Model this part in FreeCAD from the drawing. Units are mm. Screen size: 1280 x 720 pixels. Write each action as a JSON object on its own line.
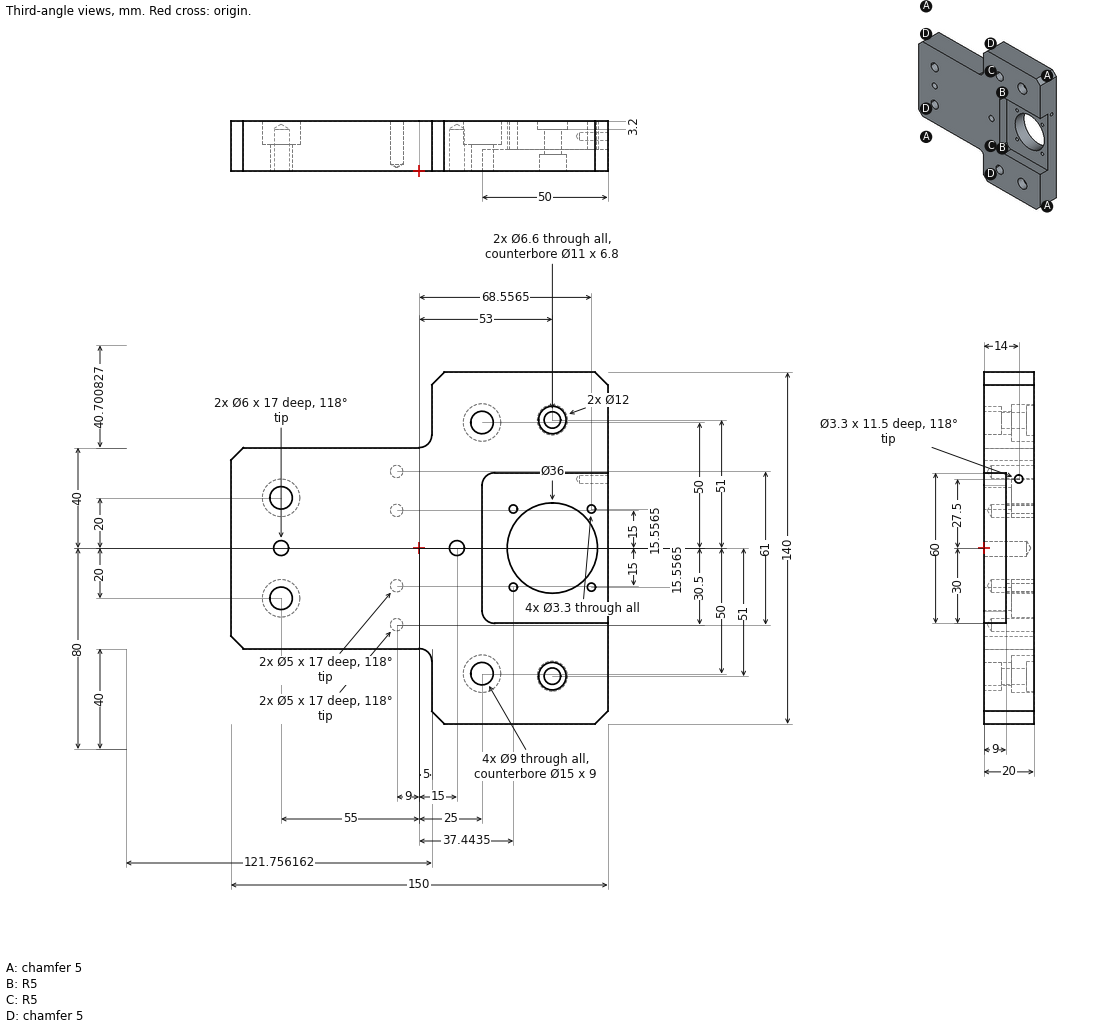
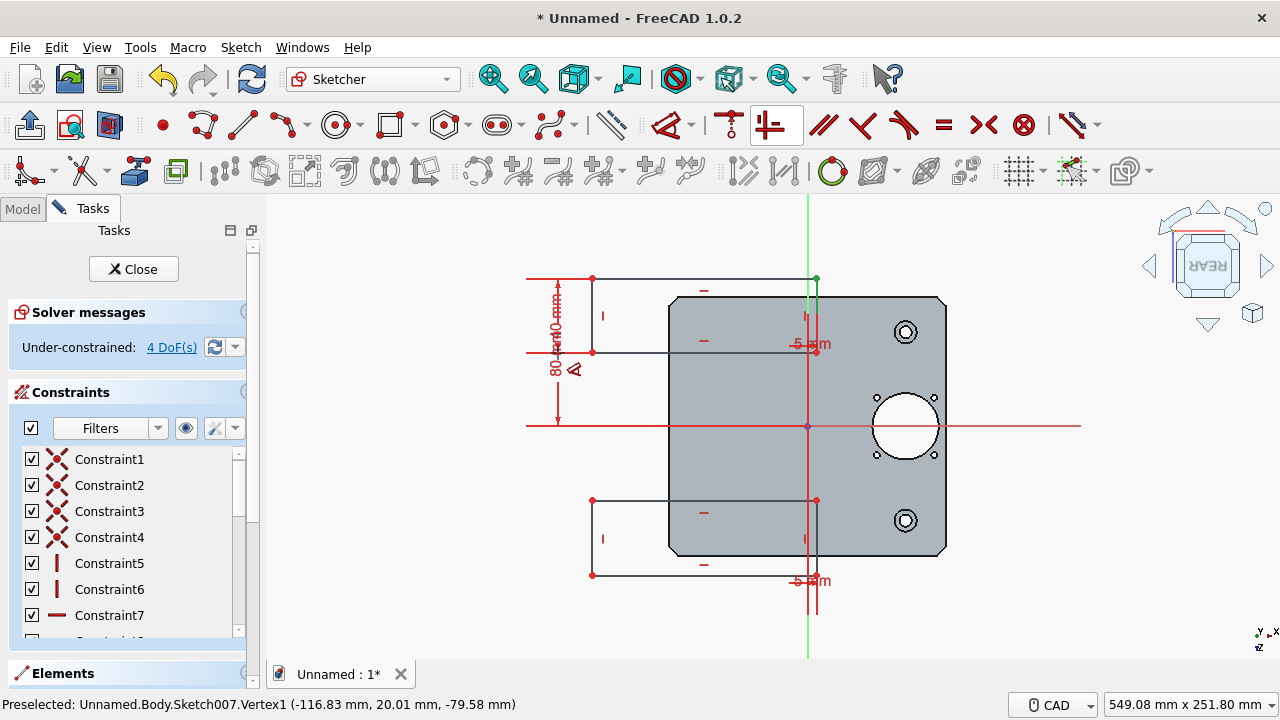
{"action": "left_click", "coordinate": [592, 501]}
{"action": "left_click", "coordinate": [558, 464]}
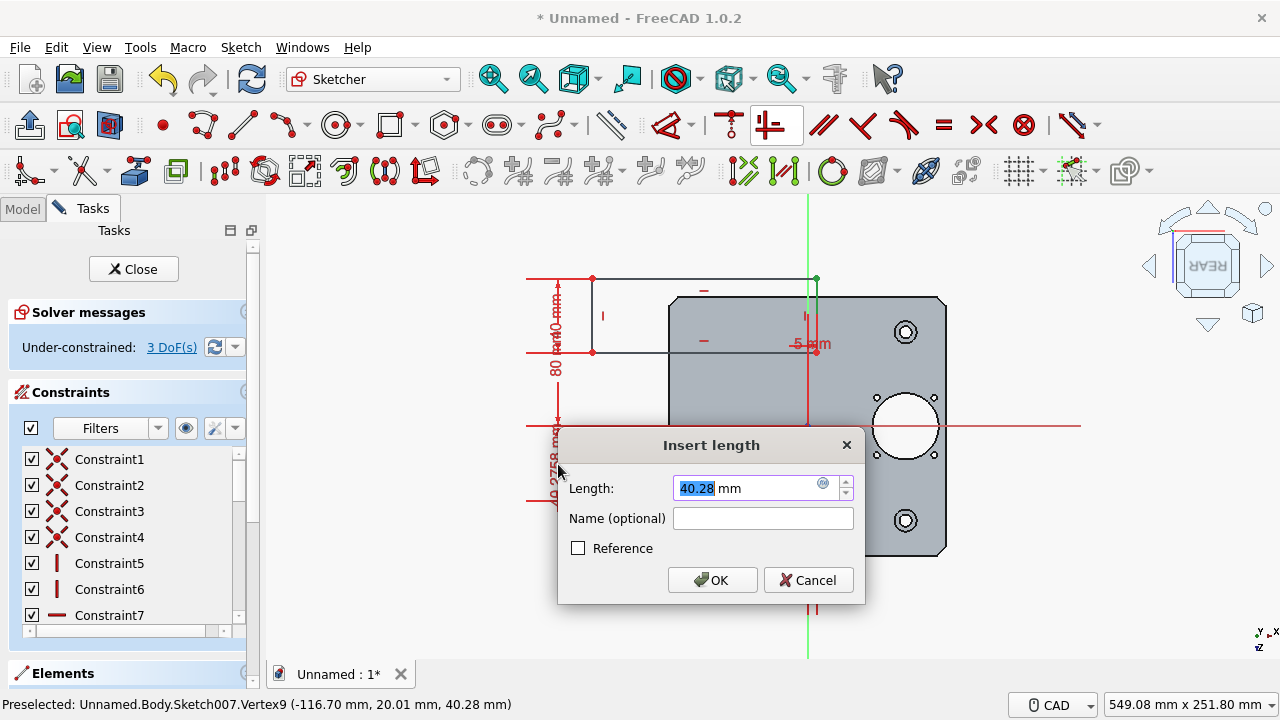
{"action": "type", "text": "40"}
{"action": "key", "text": "Return"}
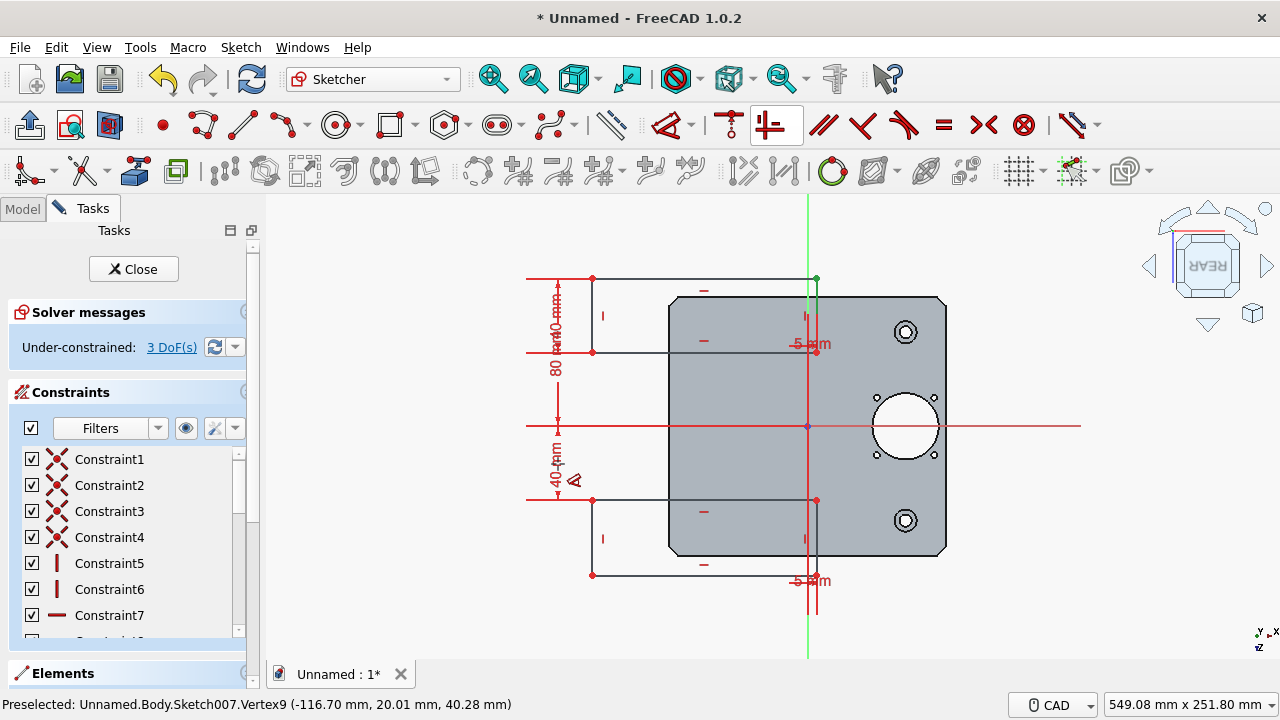
{"action": "left_click", "coordinate": [592, 523]}
{"action": "left_click", "coordinate": [558, 538]}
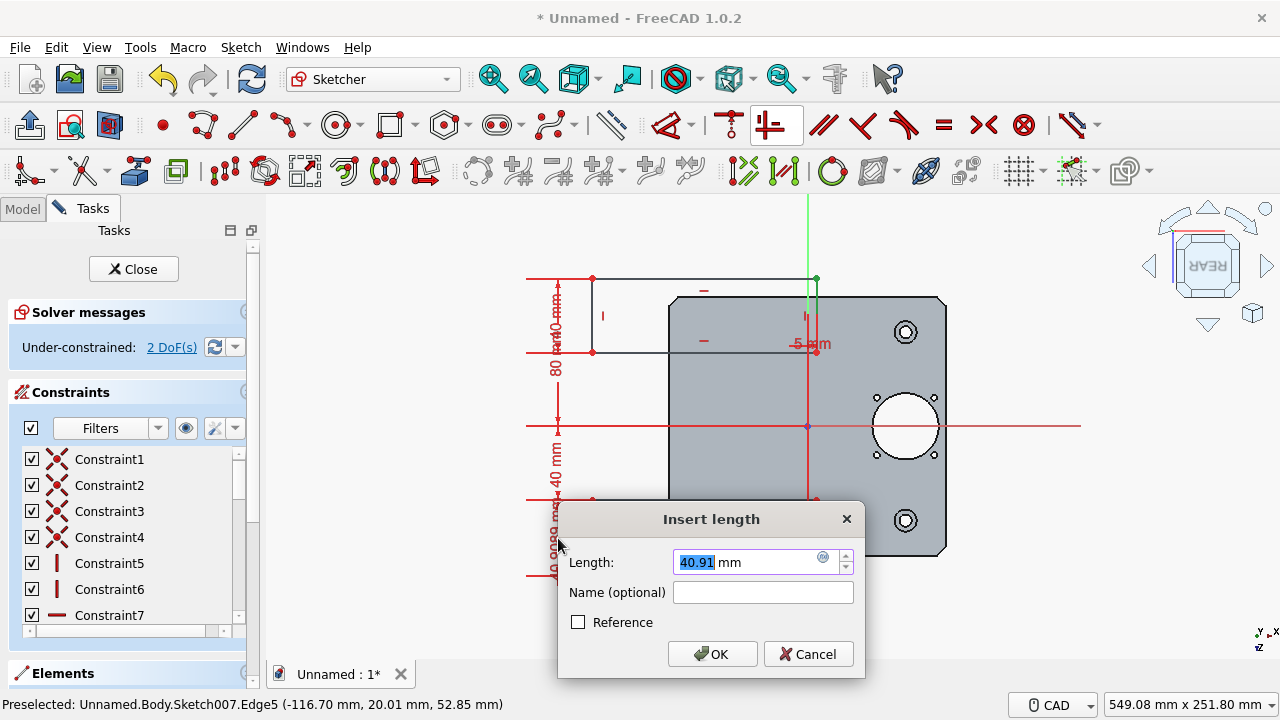
{"action": "type", "text": "40.700827"}
{"action": "key", "text": "Return"}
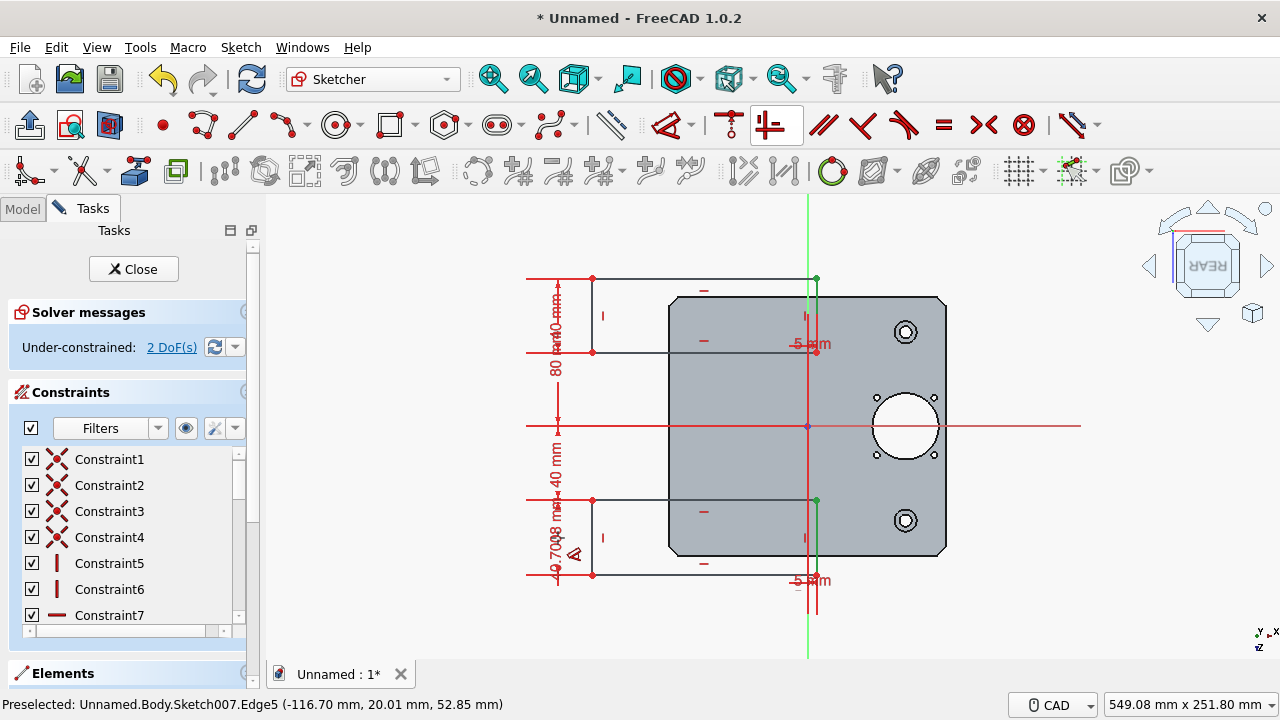
{"action": "left_click", "coordinate": [659, 353]}
{"action": "left_click", "coordinate": [704, 319]}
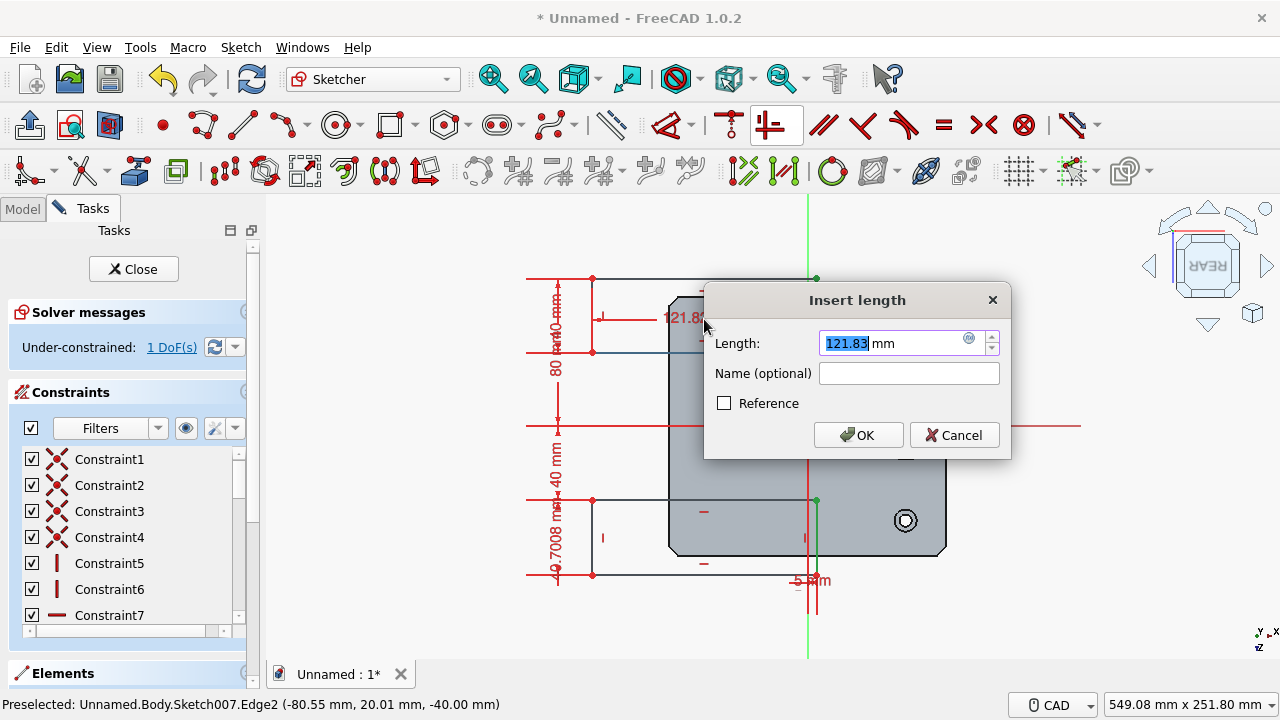
{"action": "type", "text": "121.756162"}
{"action": "key", "text": "Return"}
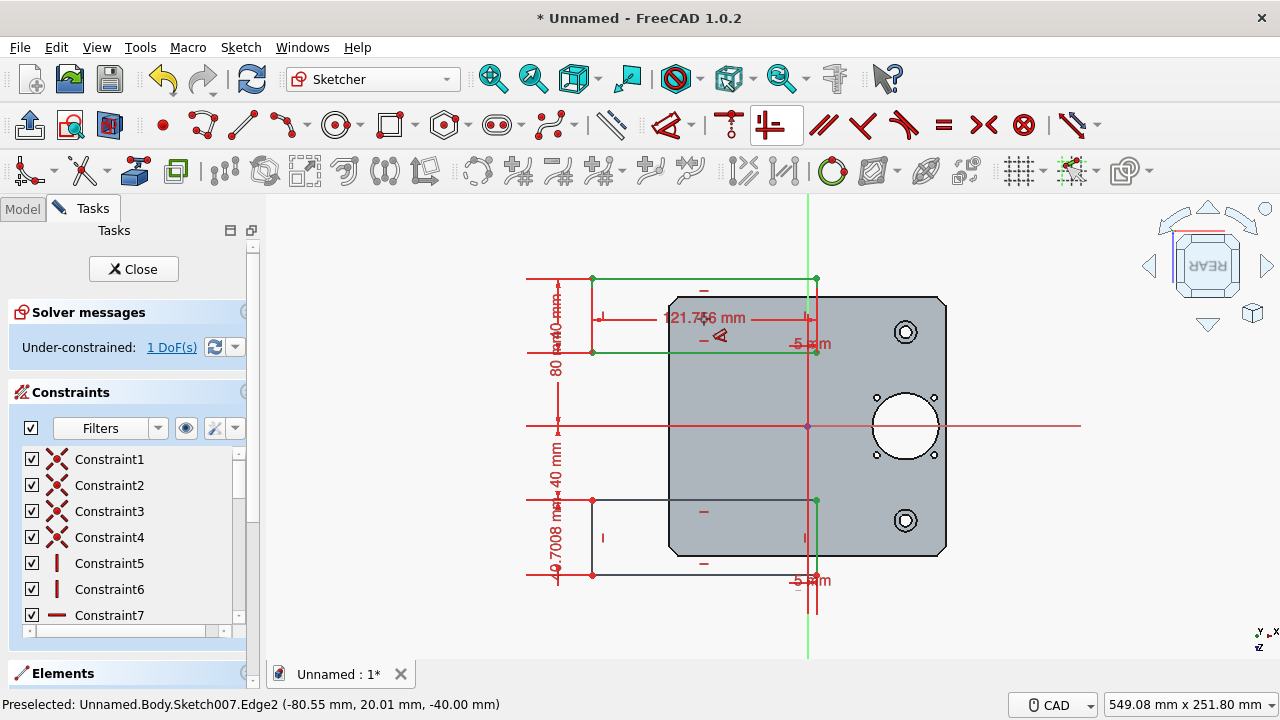
{"action": "left_click", "coordinate": [660, 575]}
{"action": "left_click", "coordinate": [705, 609]}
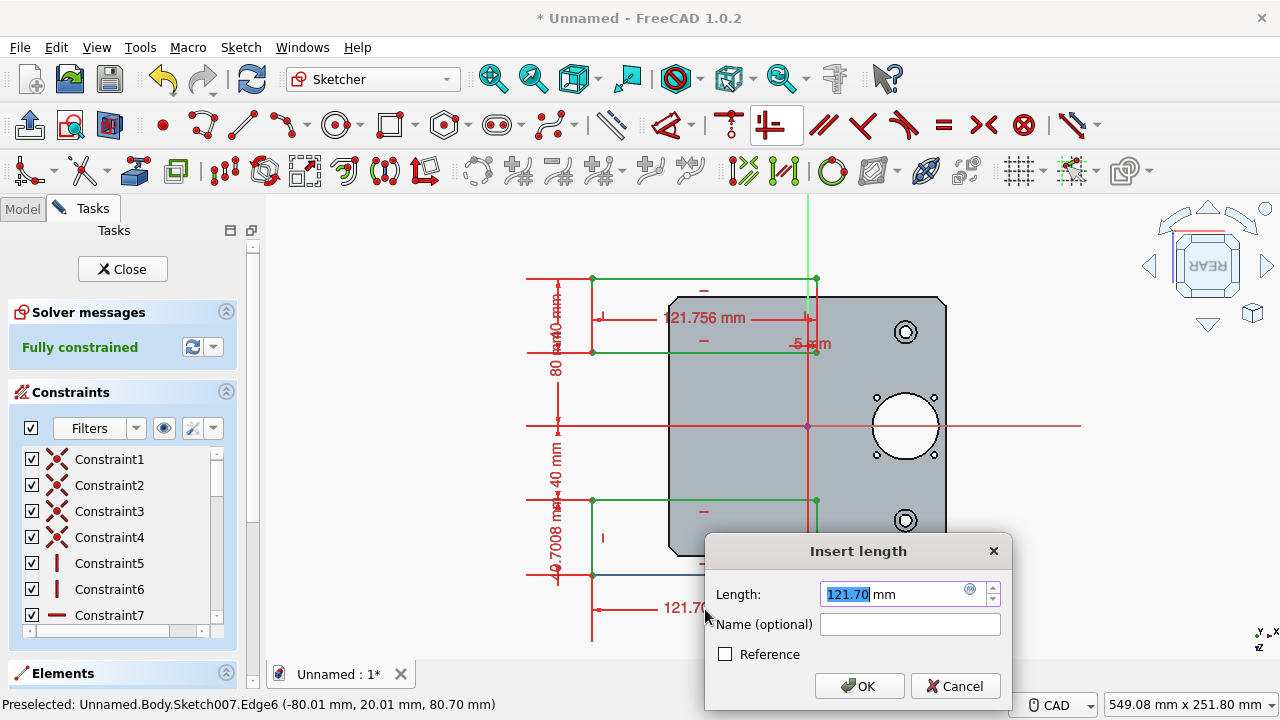
{"action": "type", "text": "121.756162"}
{"action": "key", "text": "Return"}
{"action": "key", "text": "Escape"}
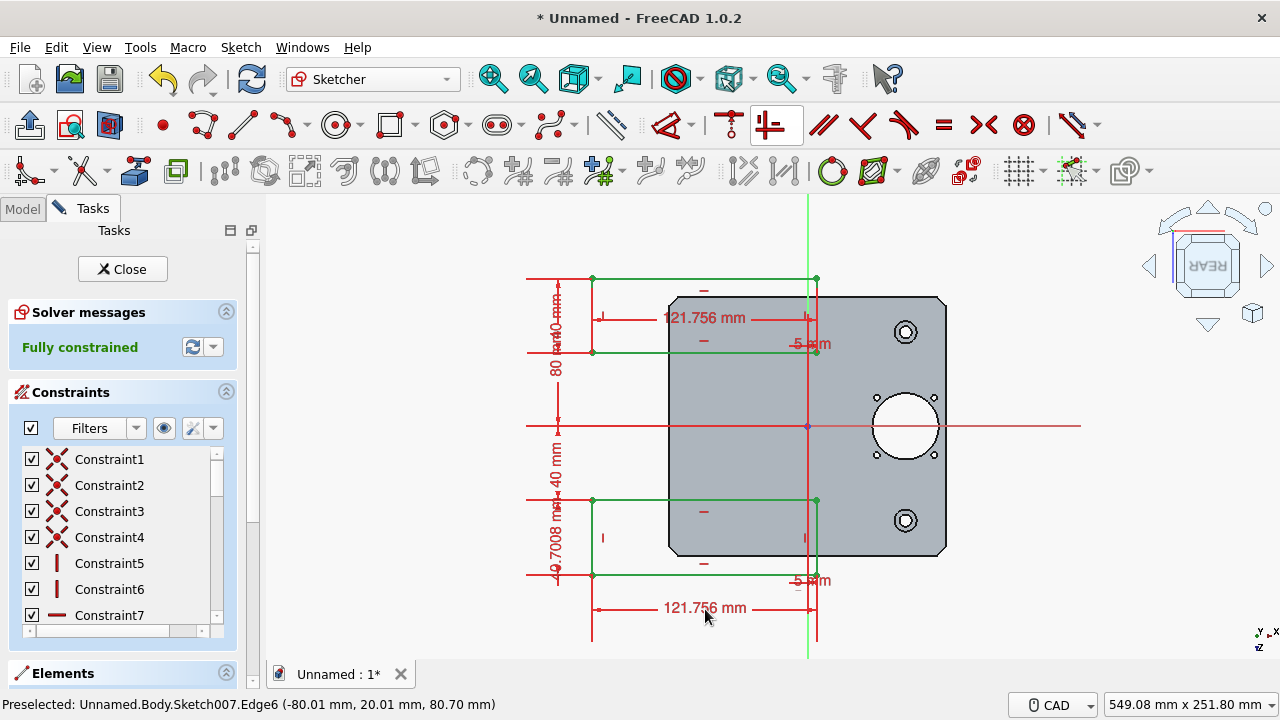
{"action": "left_click", "coordinate": [123, 269]}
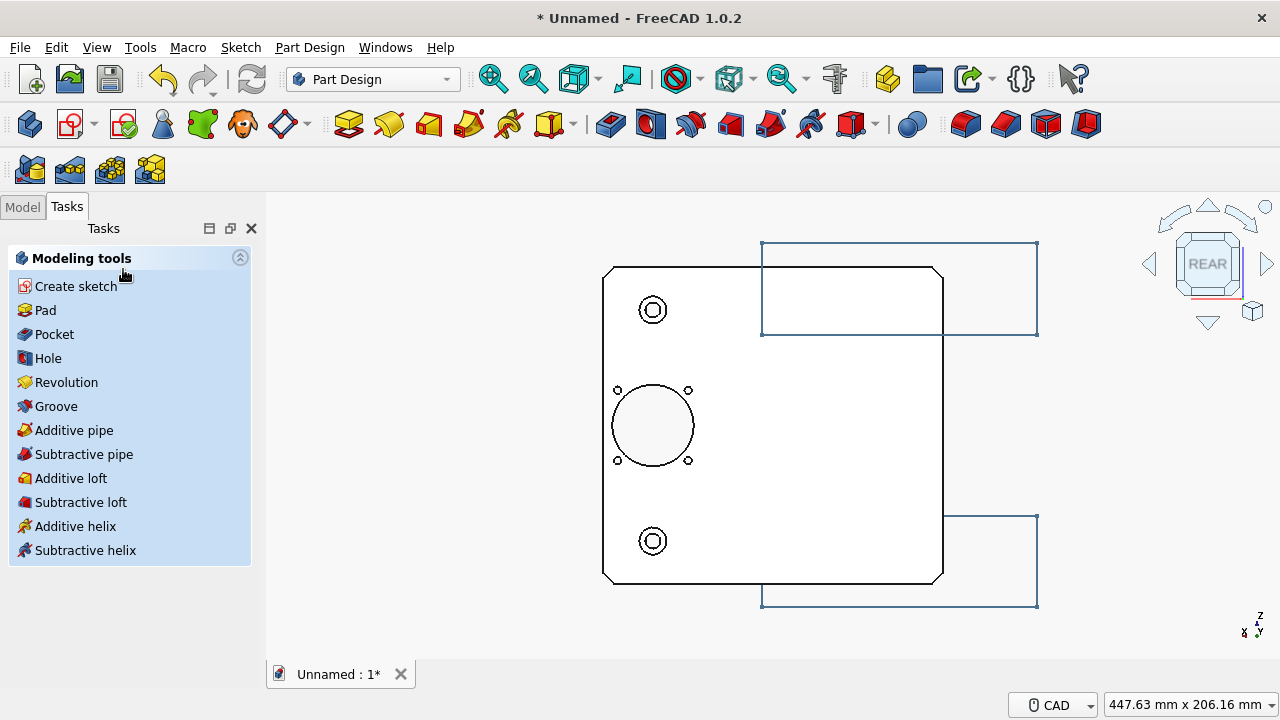
{"action": "left_click", "coordinate": [612, 124]}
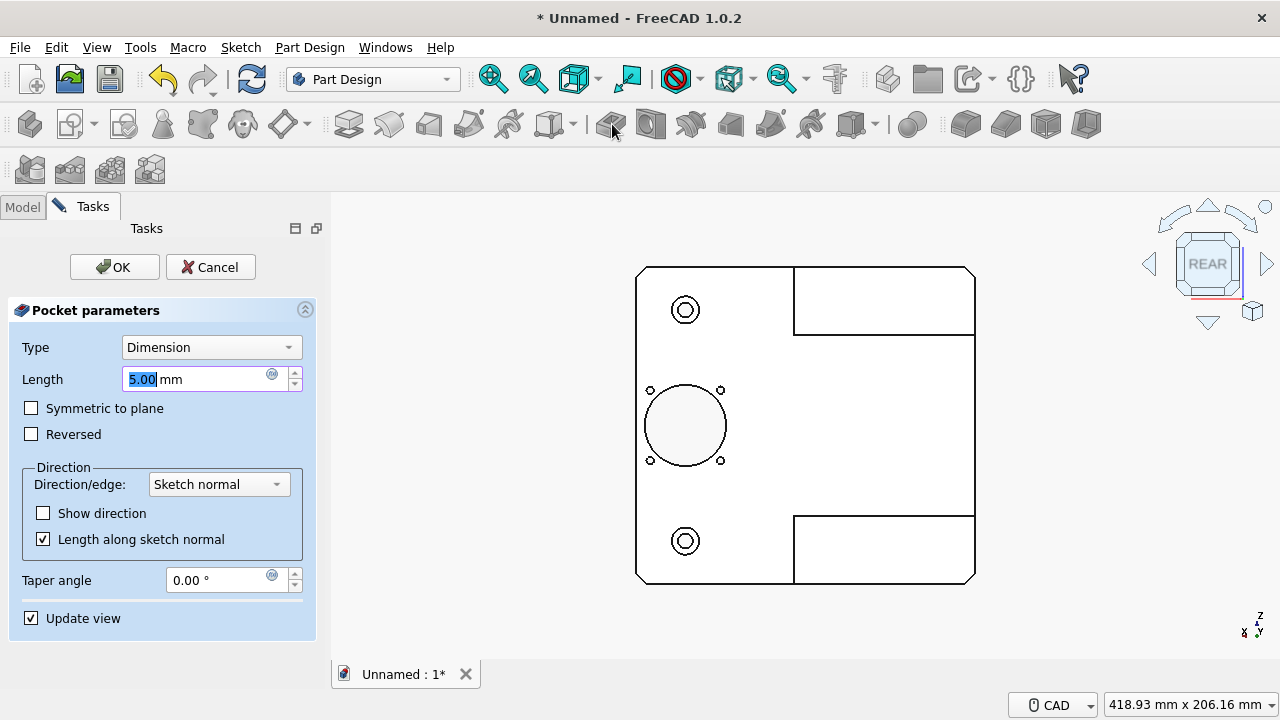
{"action": "left_click", "coordinate": [212, 348]}